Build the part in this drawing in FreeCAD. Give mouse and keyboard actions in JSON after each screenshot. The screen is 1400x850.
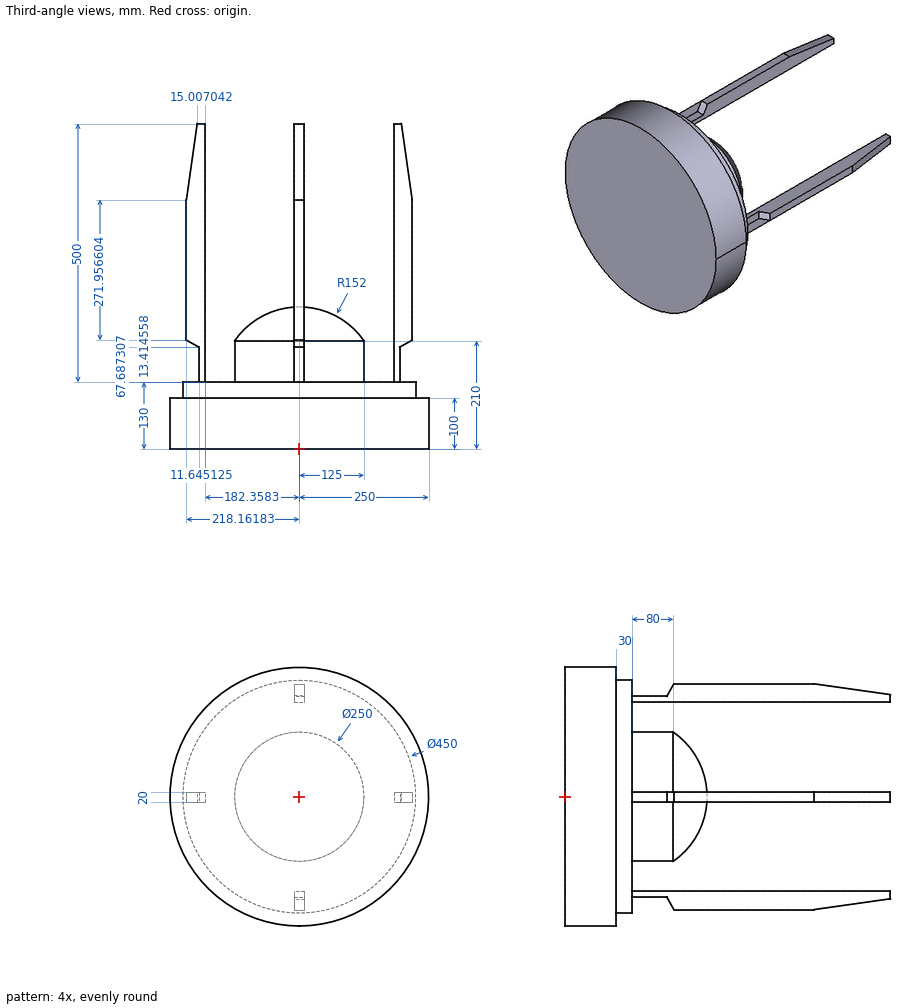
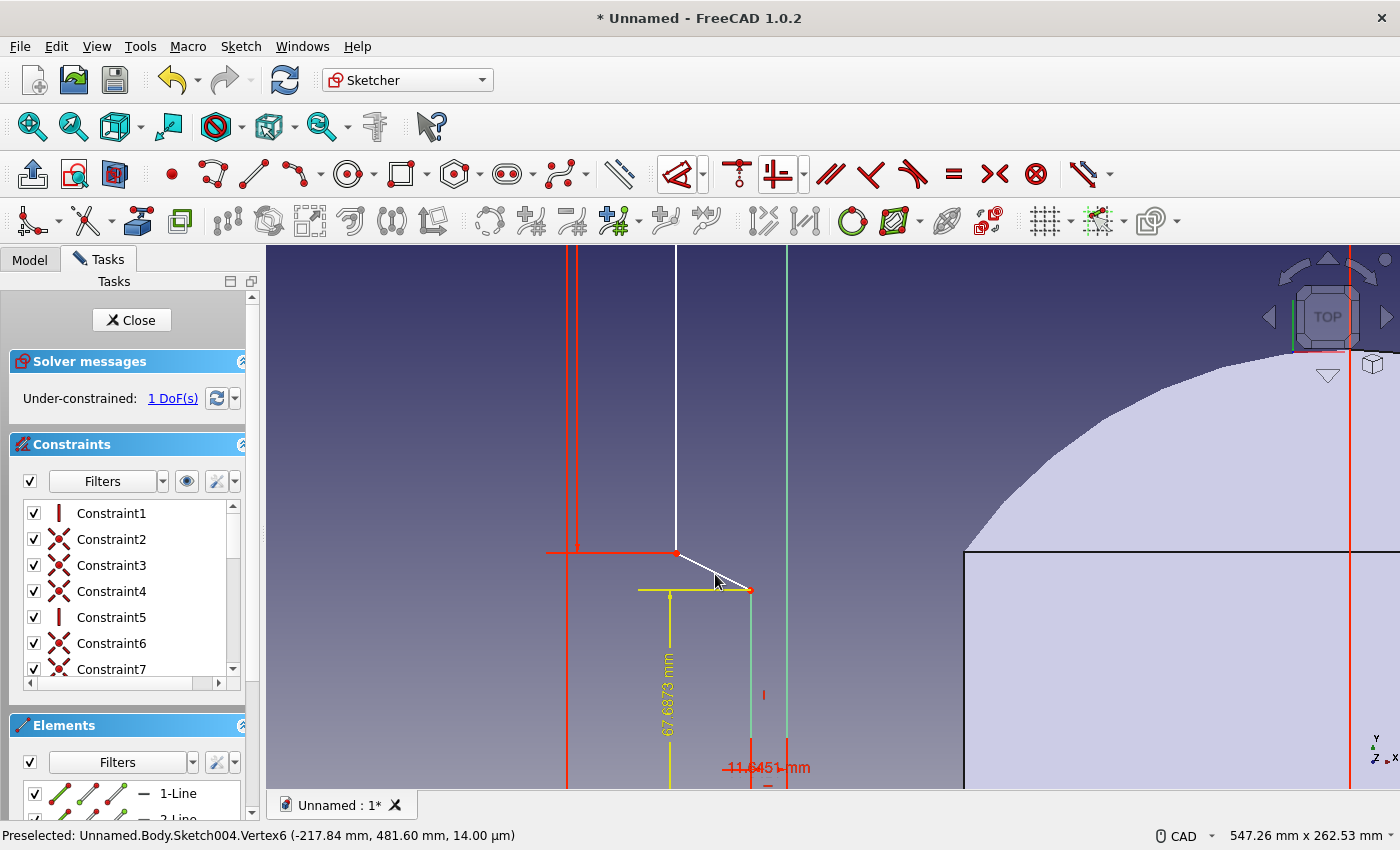
{"action": "left_click", "coordinate": [713, 572]}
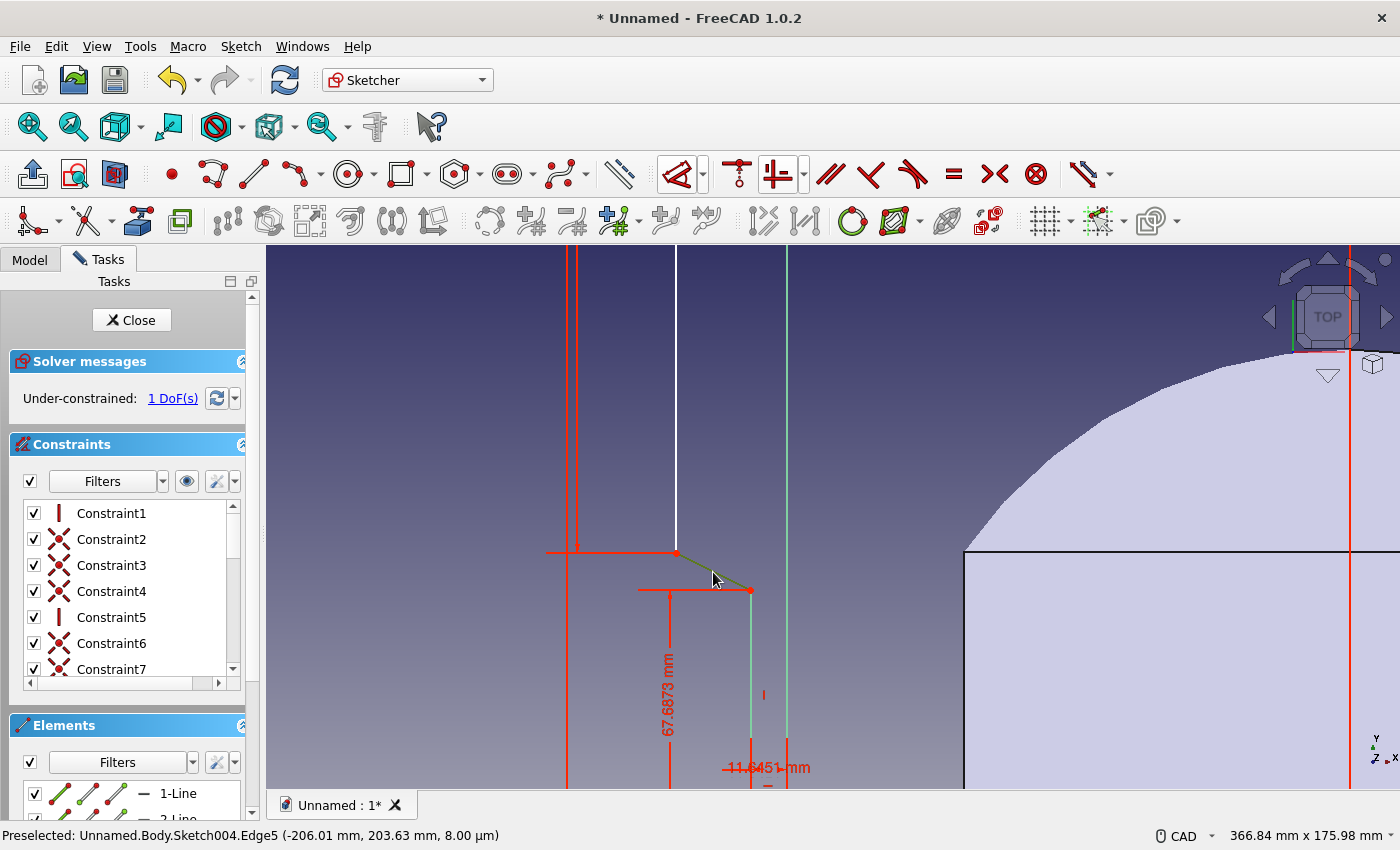
{"action": "left_click", "coordinate": [702, 174]}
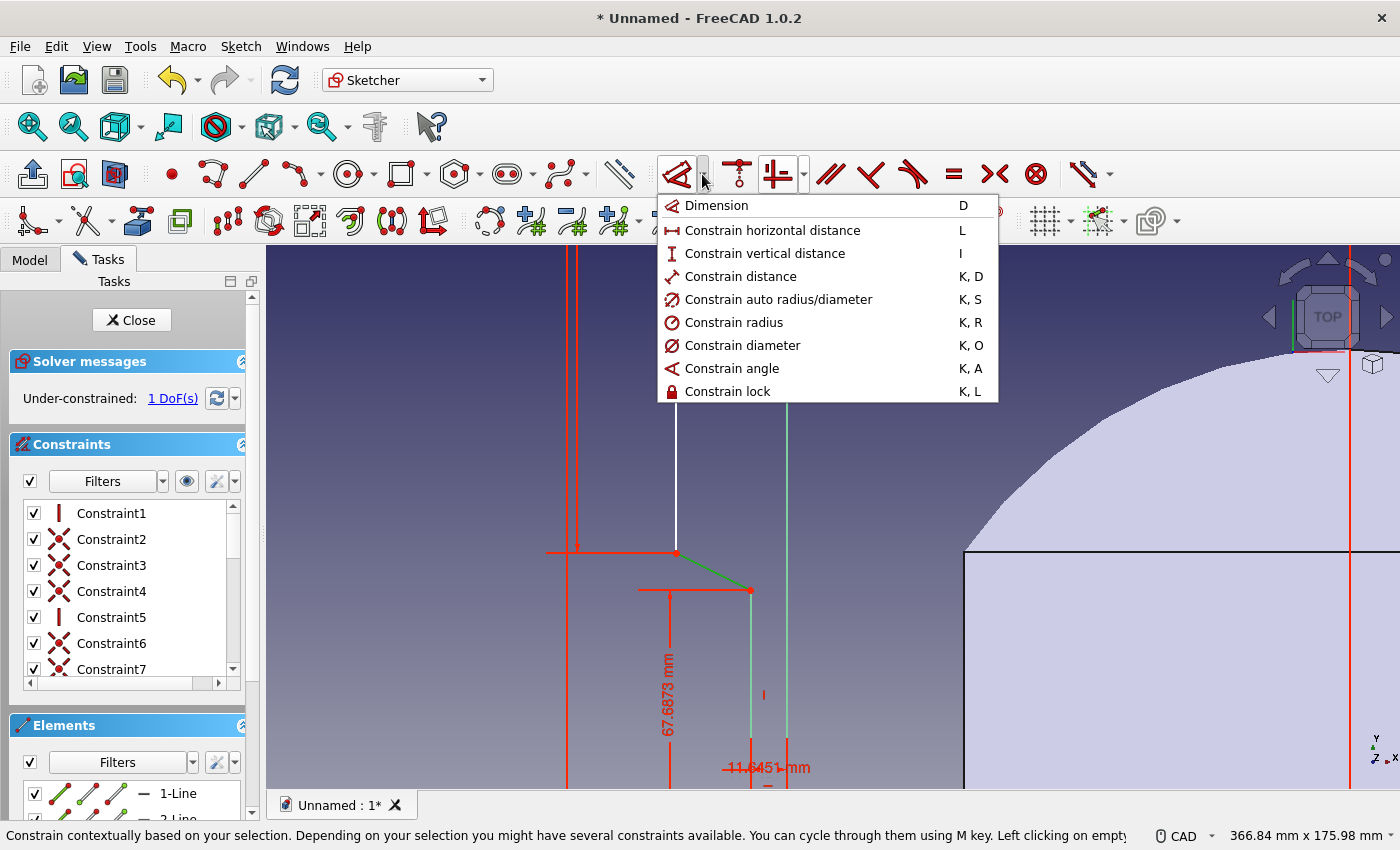
{"action": "left_click", "coordinate": [828, 254]}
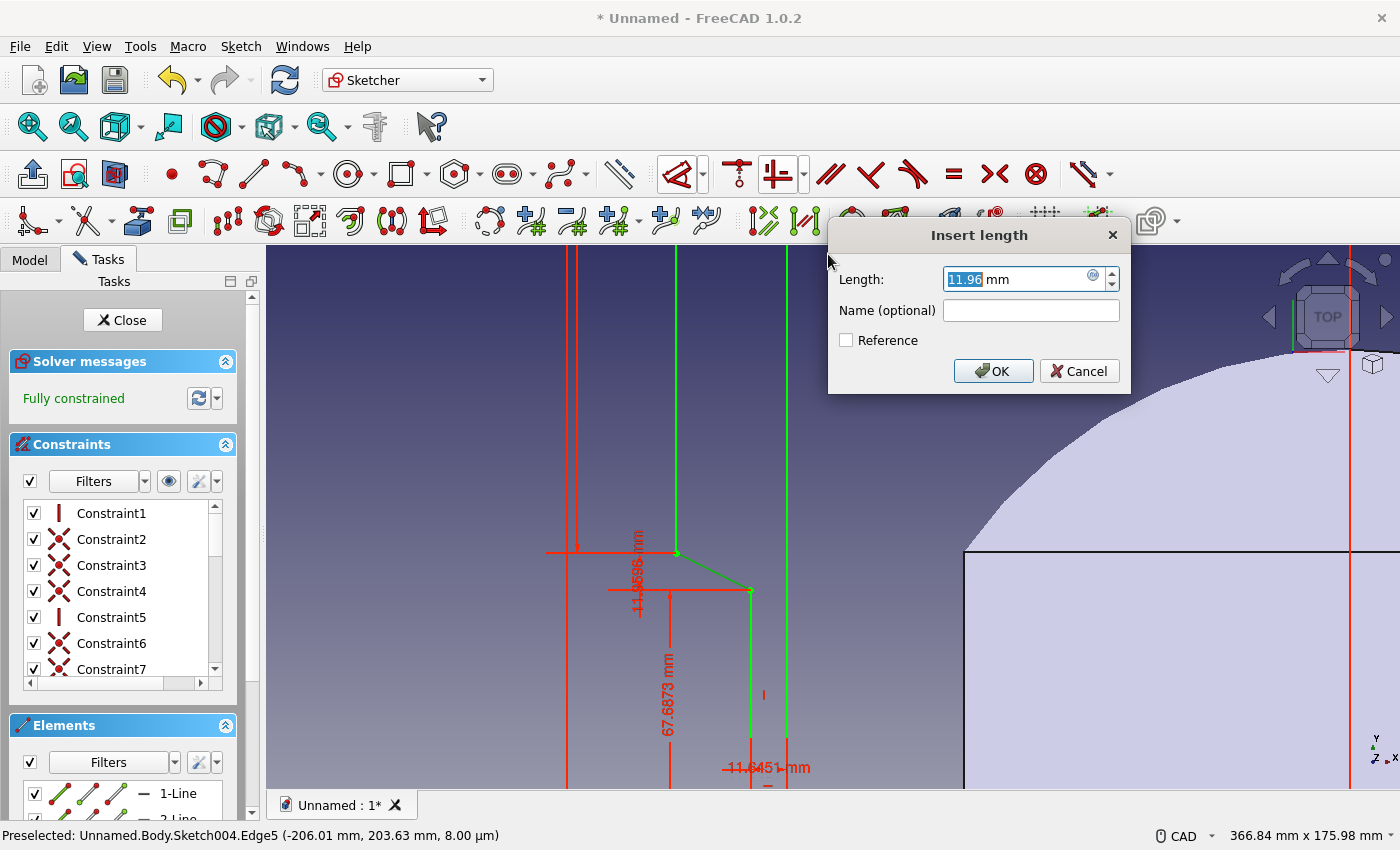
{"action": "type", "text": "13.414558"}
{"action": "key", "text": "Return"}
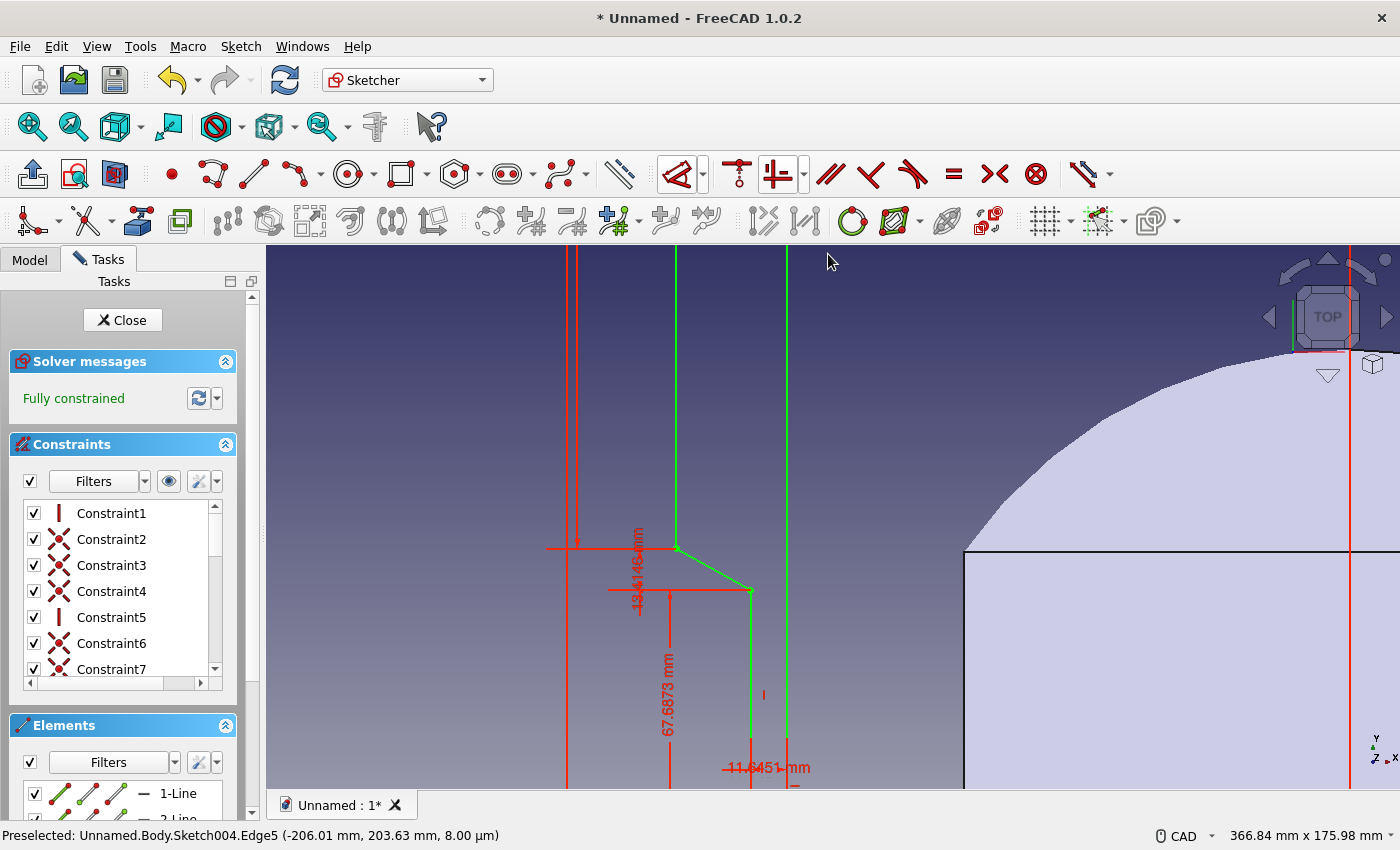
{"action": "left_click", "coordinate": [123, 320]}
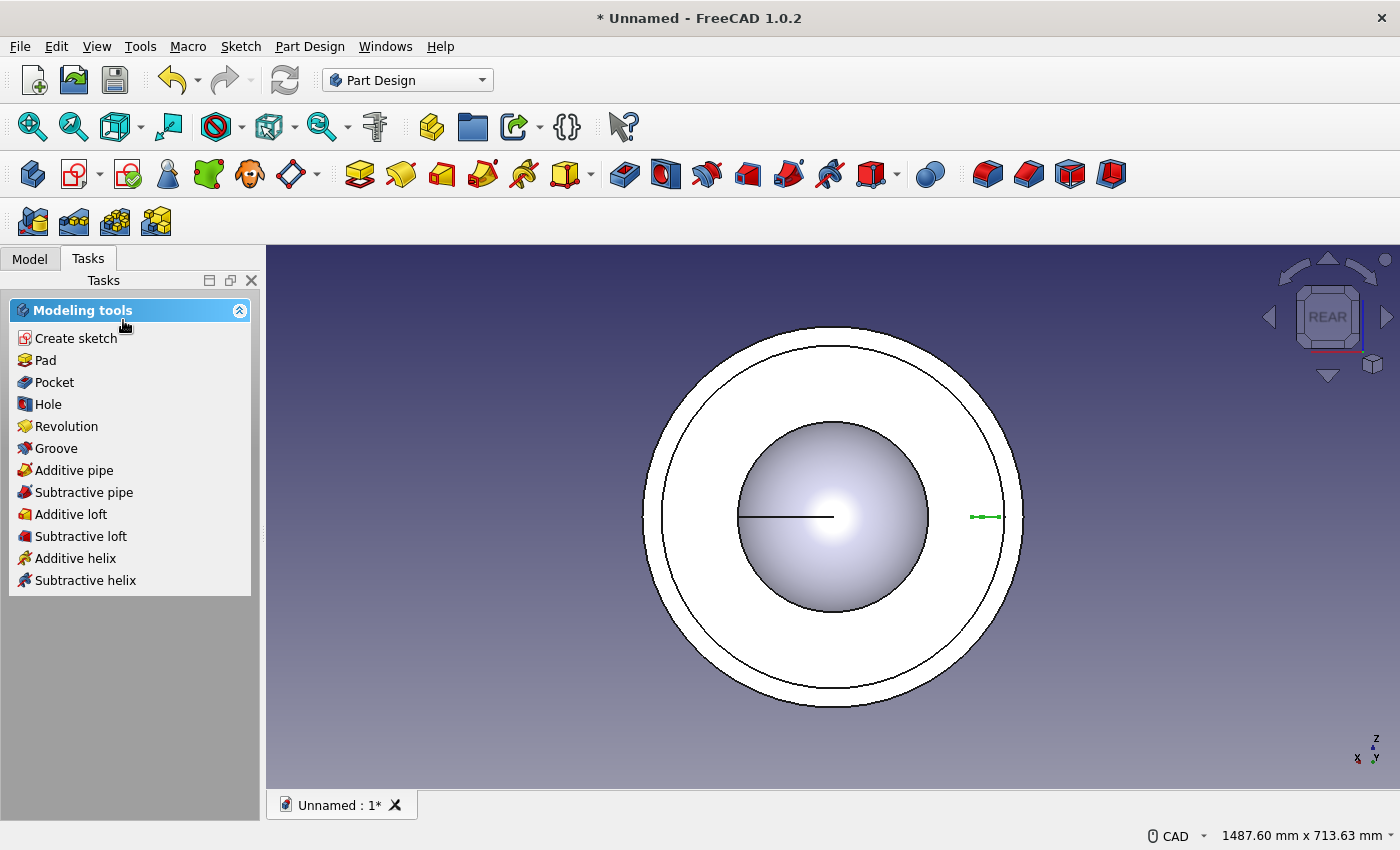
{"action": "left_click", "coordinate": [360, 174]}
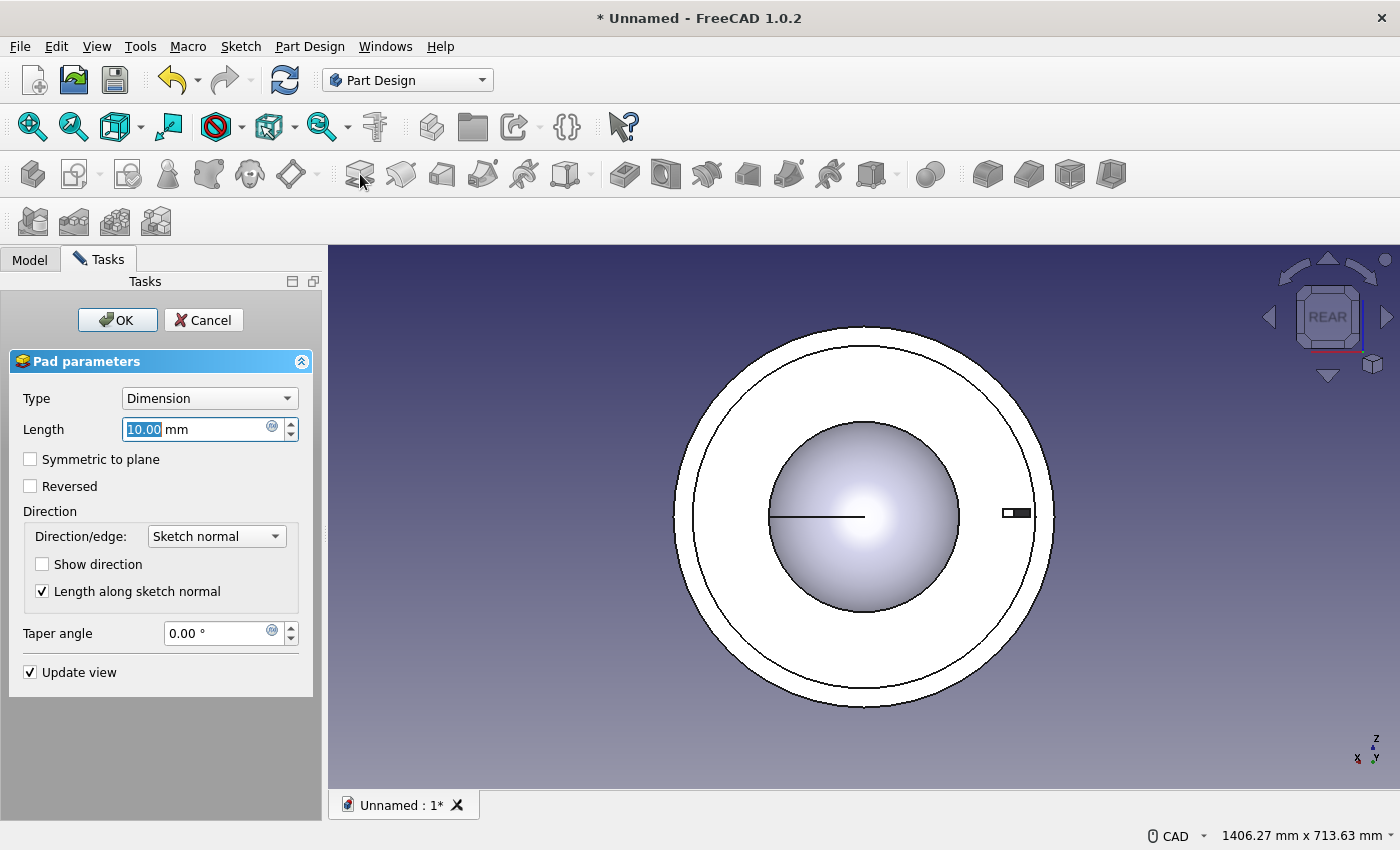
{"action": "type", "text": "20"}
{"action": "key", "text": "Tab"}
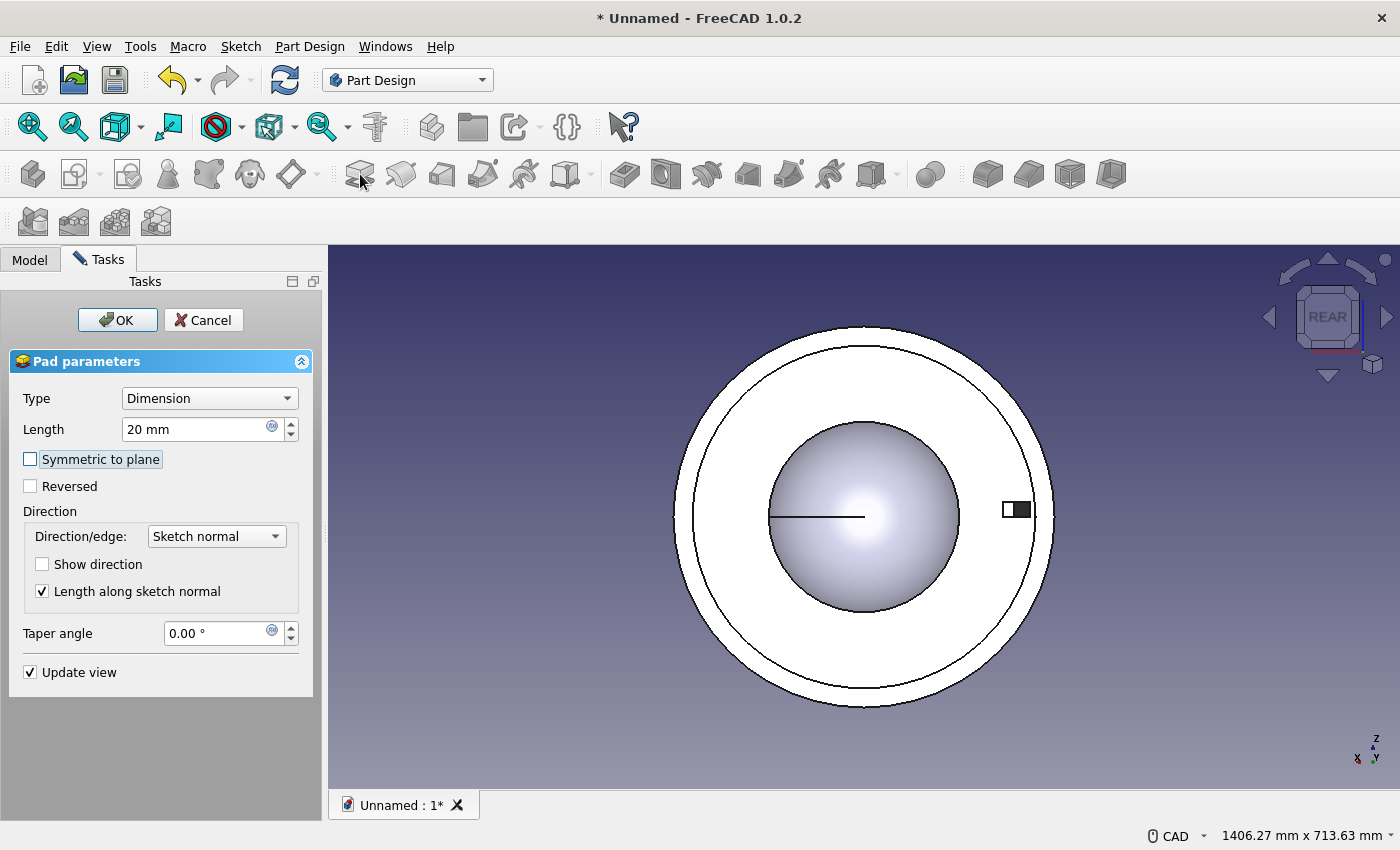
{"action": "left_click", "coordinate": [31, 459]}